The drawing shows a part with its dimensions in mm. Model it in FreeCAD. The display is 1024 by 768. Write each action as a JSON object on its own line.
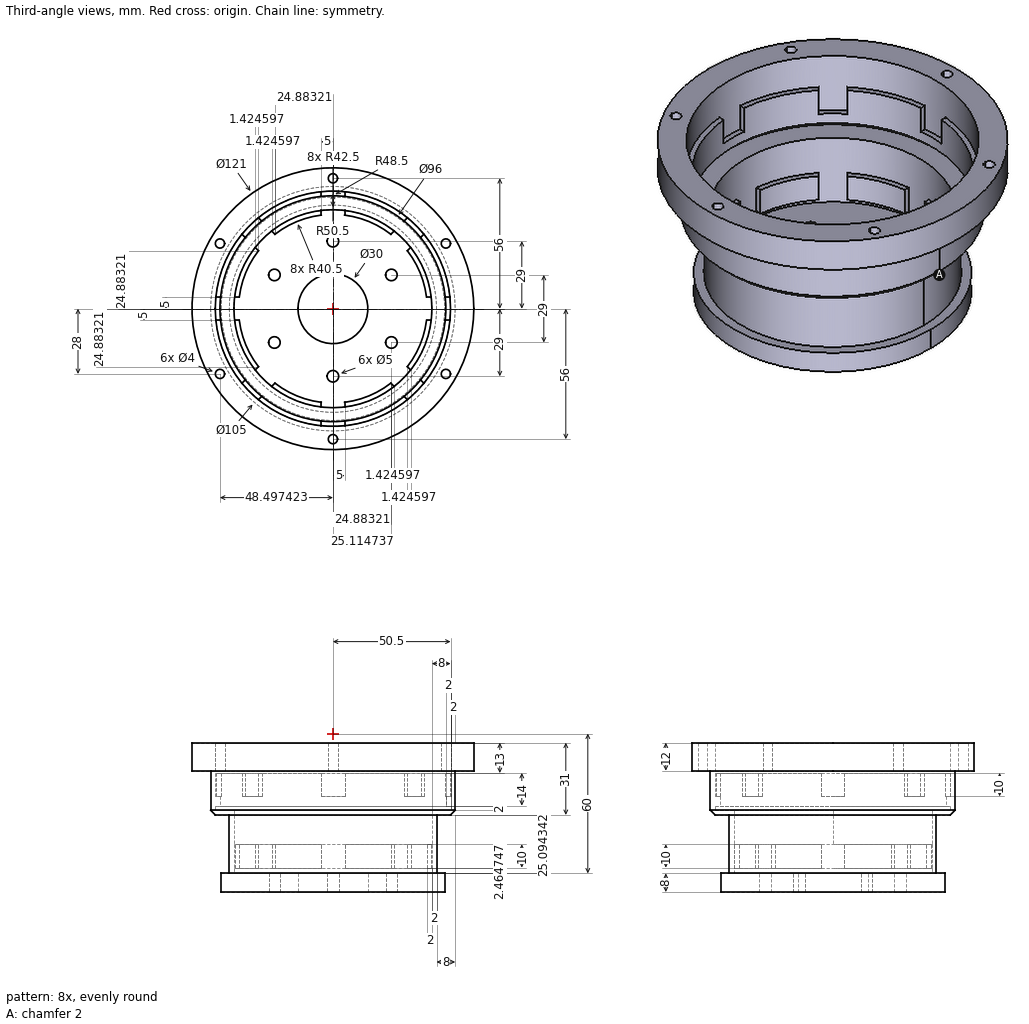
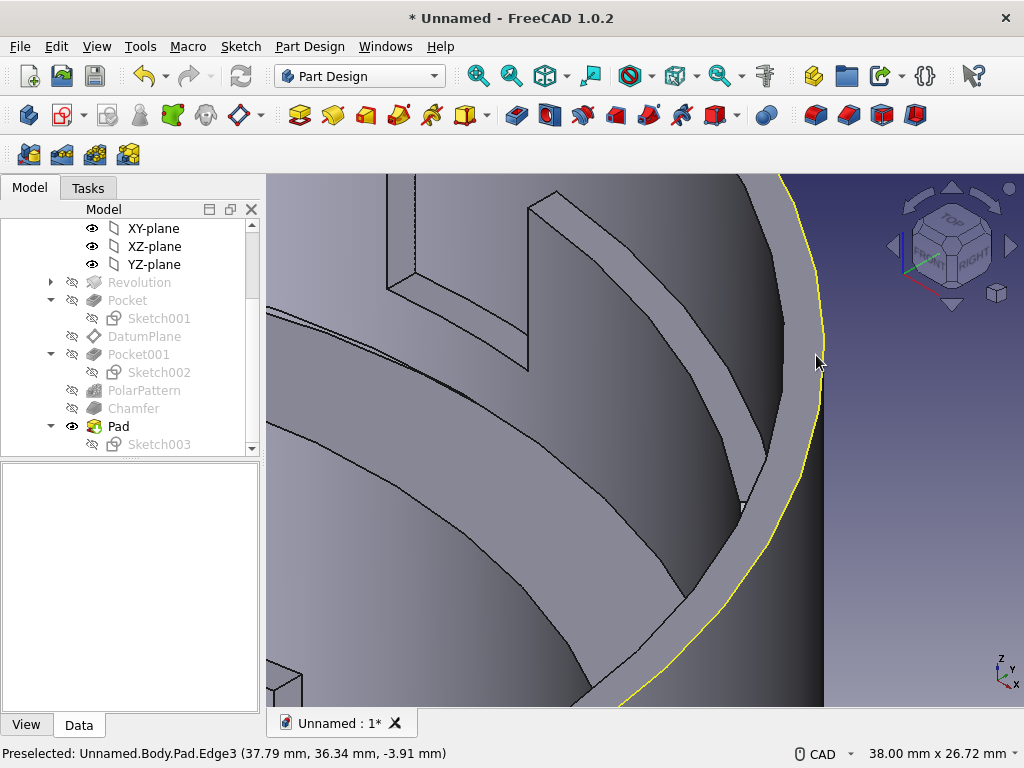
{"action": "left_click", "coordinate": [811, 360]}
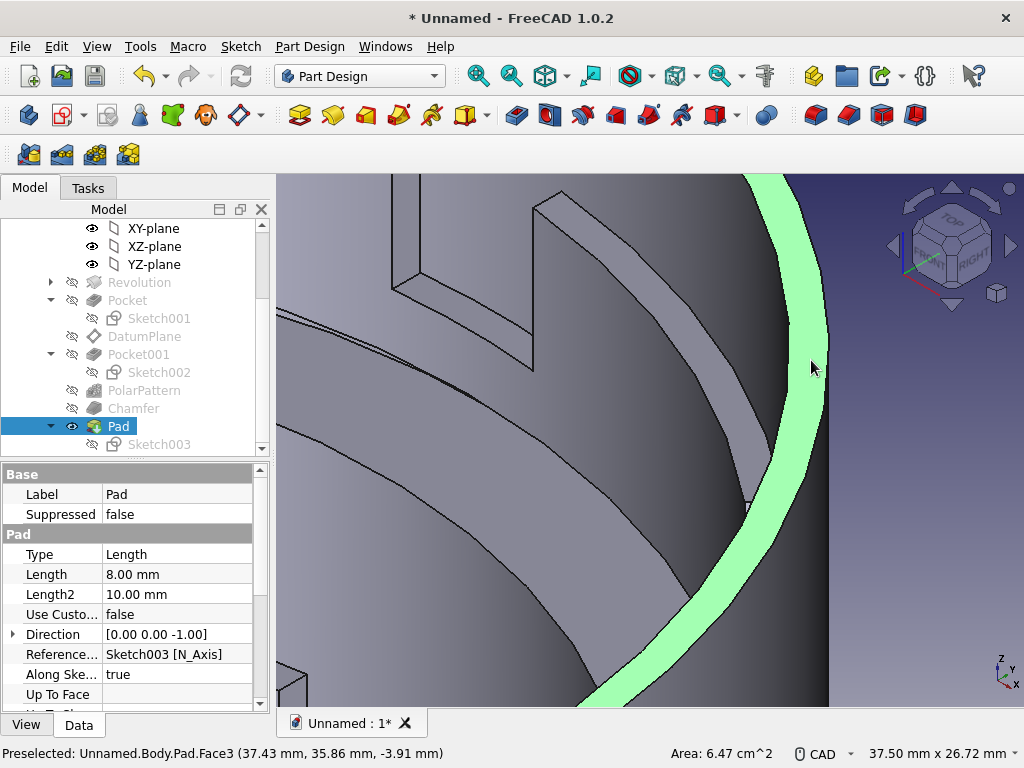
{"action": "left_click", "coordinate": [62, 116]}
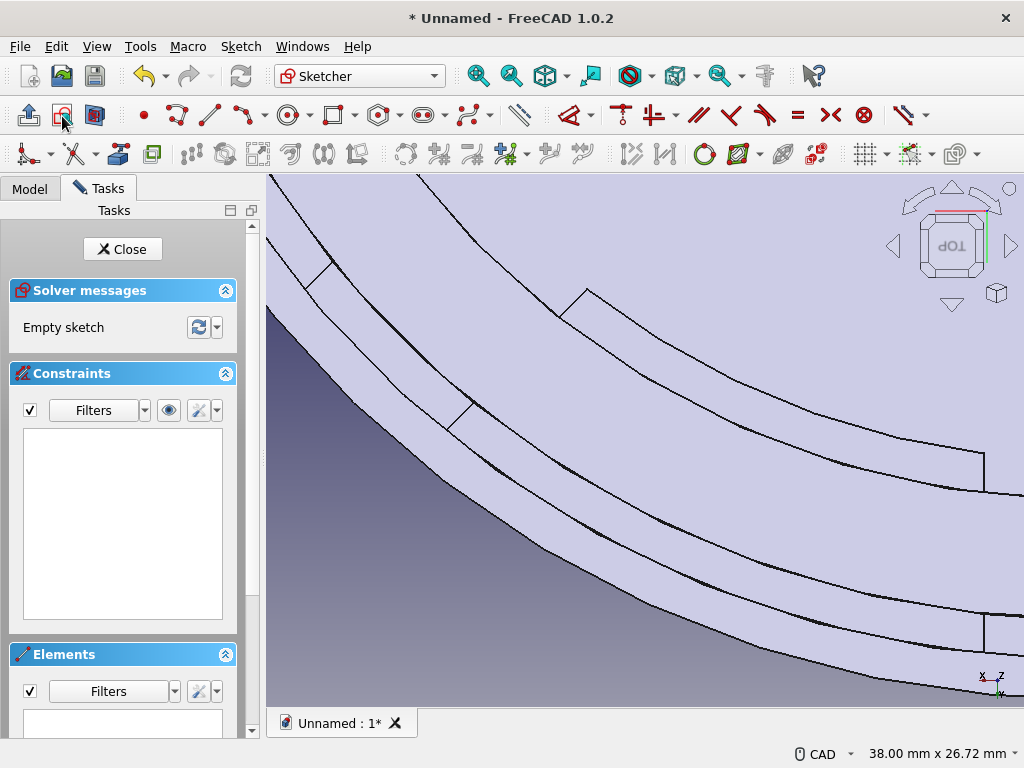
{"action": "scroll", "coordinate": [497, 564], "scroll_direction": "down", "scroll_amount": 10}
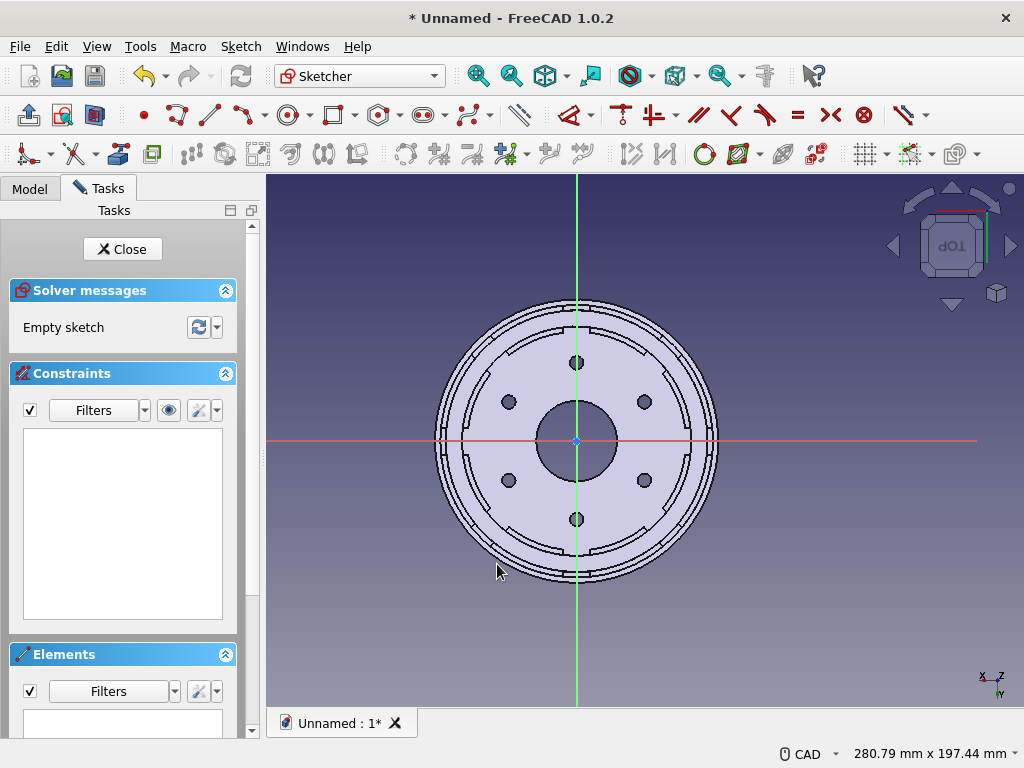
{"action": "left_click", "coordinate": [288, 116]}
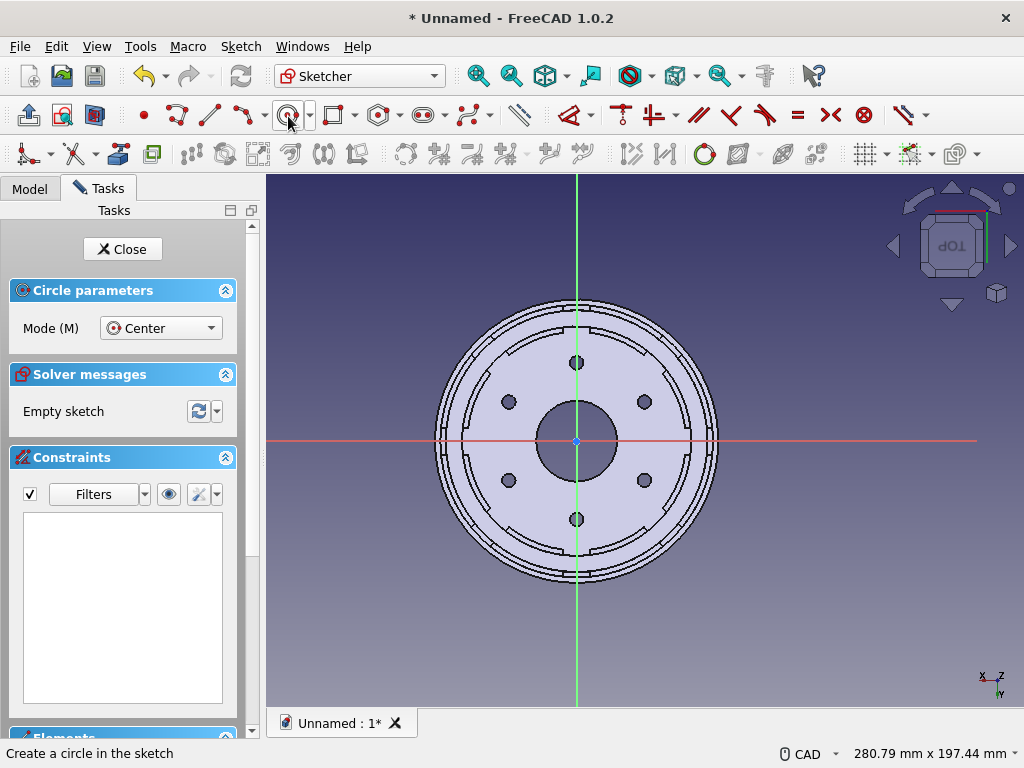
{"action": "left_click", "coordinate": [577, 441]}
{"action": "left_click", "coordinate": [692, 326]}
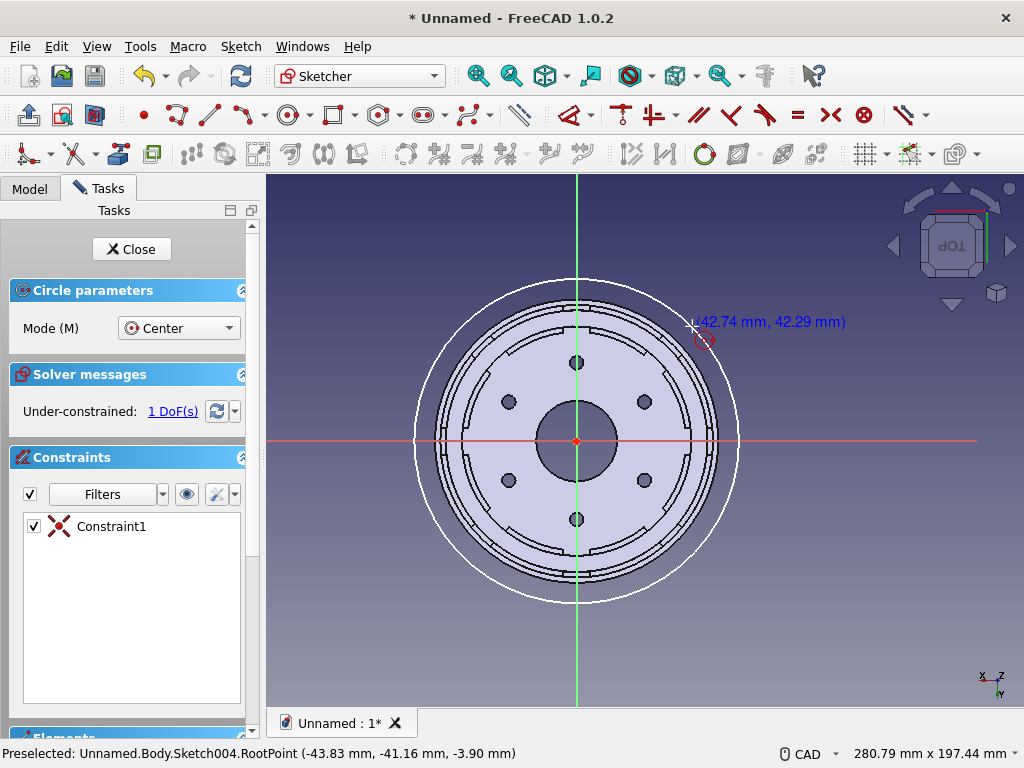
{"action": "scroll", "coordinate": [708, 366], "scroll_direction": "up", "scroll_amount": 8}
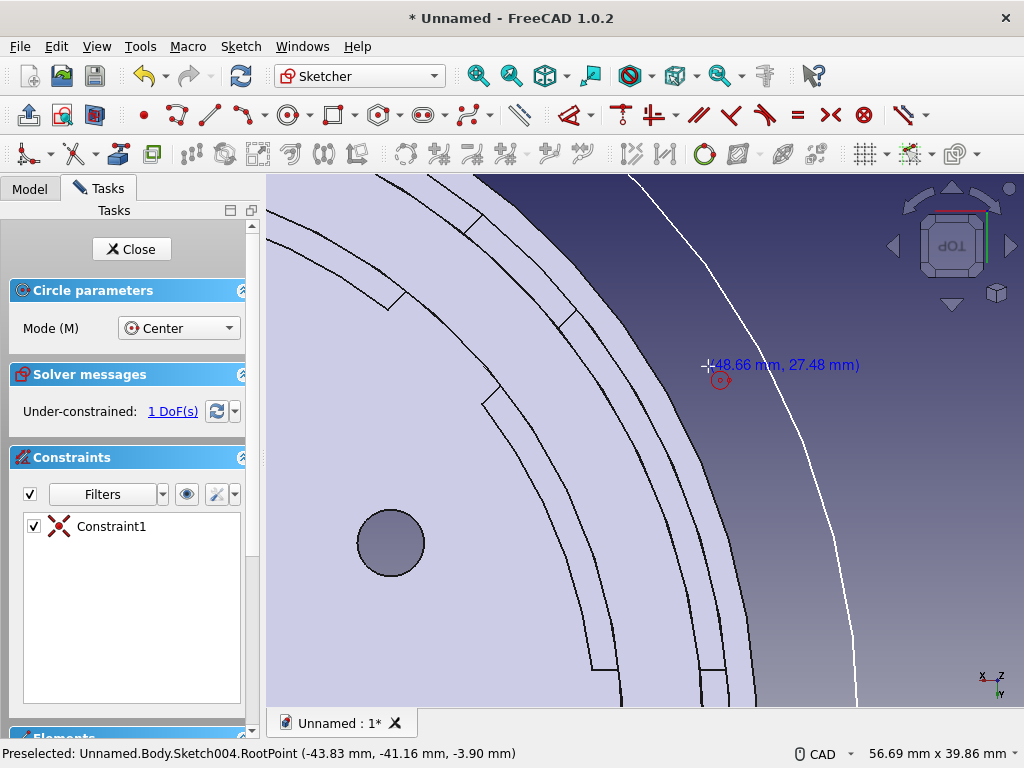
{"action": "scroll", "coordinate": [708, 366], "scroll_direction": "down", "scroll_amount": 8}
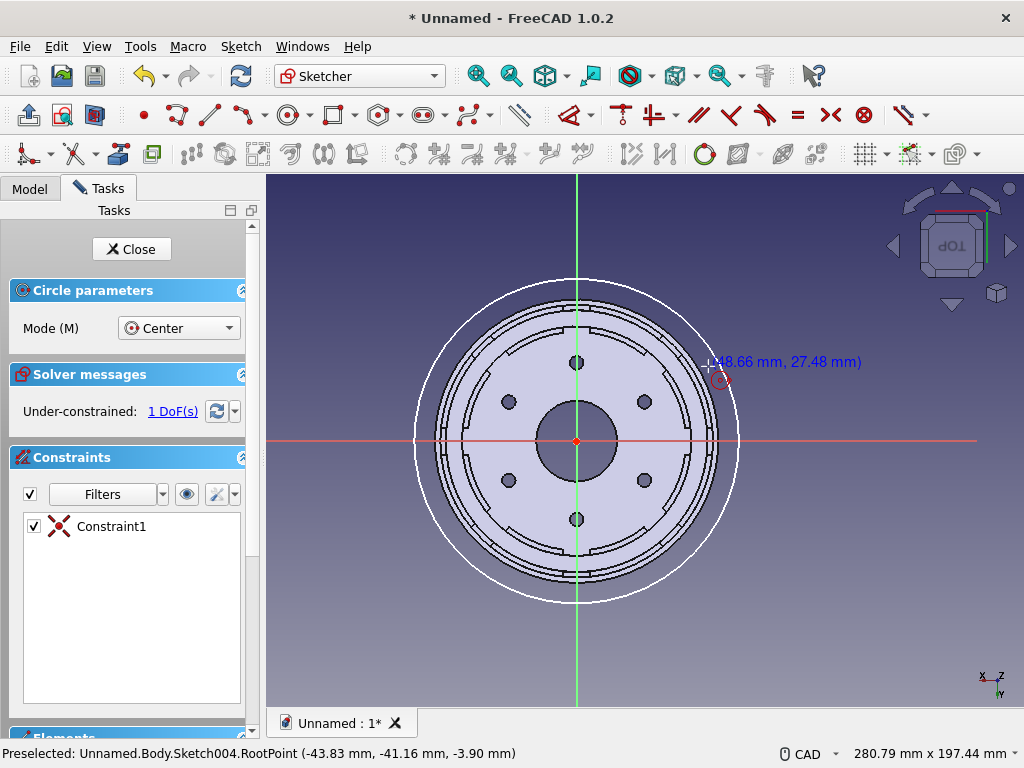
{"action": "scroll", "coordinate": [708, 366], "scroll_direction": "up", "scroll_amount": 2}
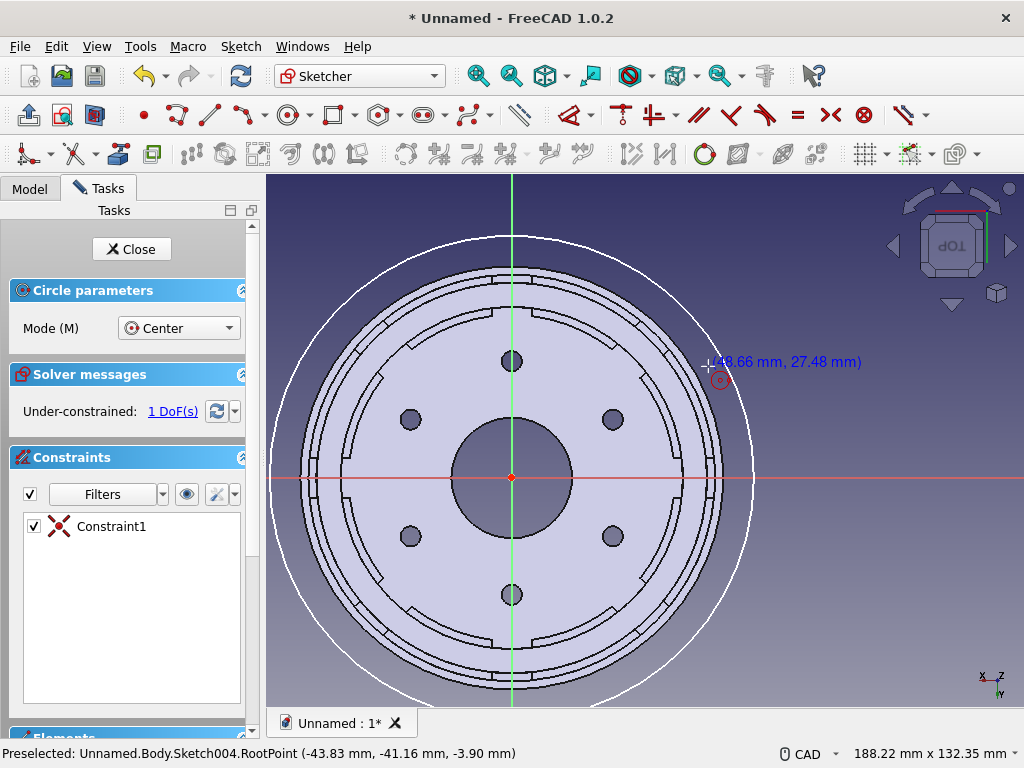
{"action": "left_click", "coordinate": [707, 365]}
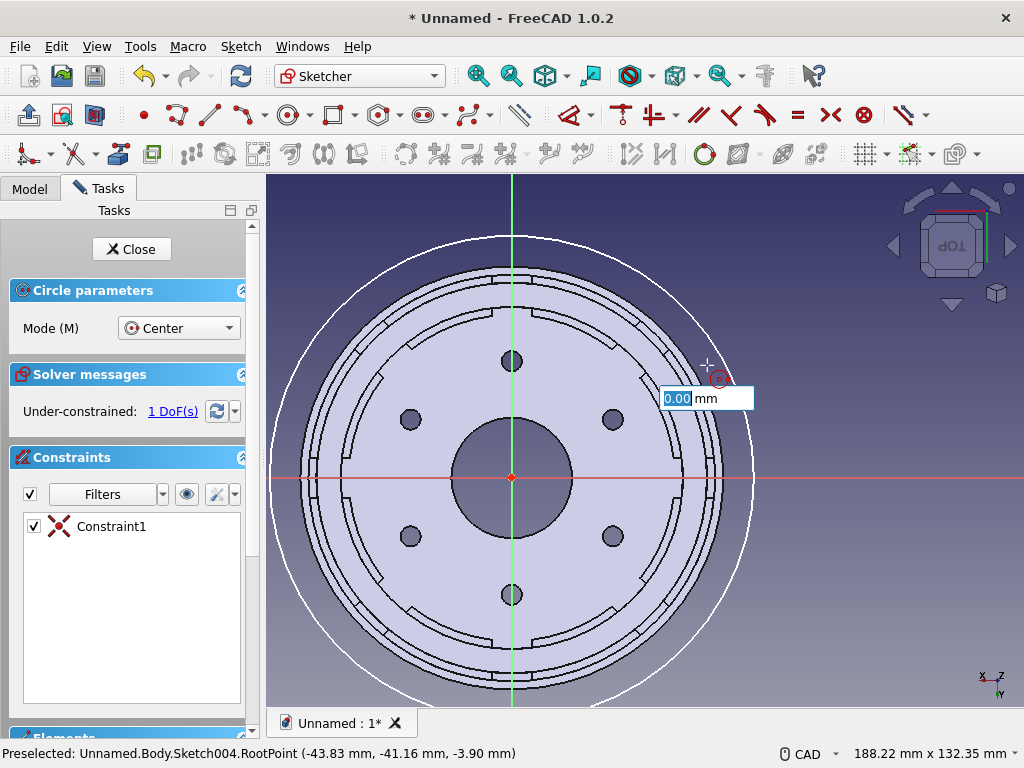
{"action": "scroll", "coordinate": [701, 360], "scroll_direction": "up", "scroll_amount": 4}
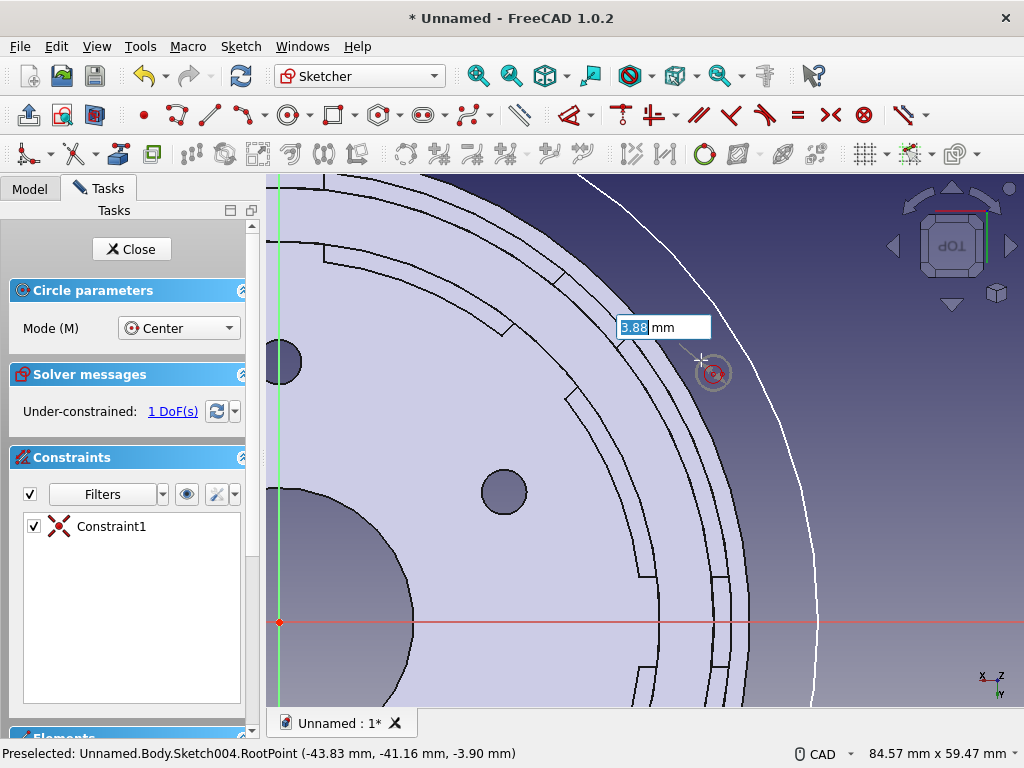
{"action": "left_click", "coordinate": [701, 358]}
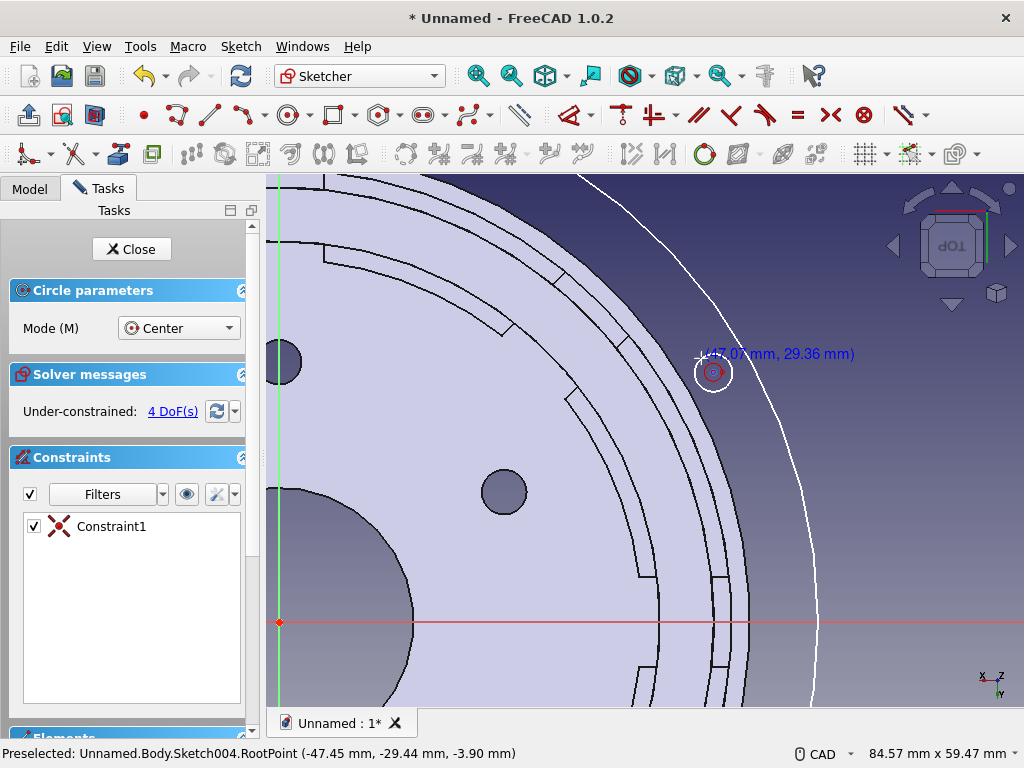
{"action": "scroll", "coordinate": [705, 362], "scroll_direction": "down", "scroll_amount": 6}